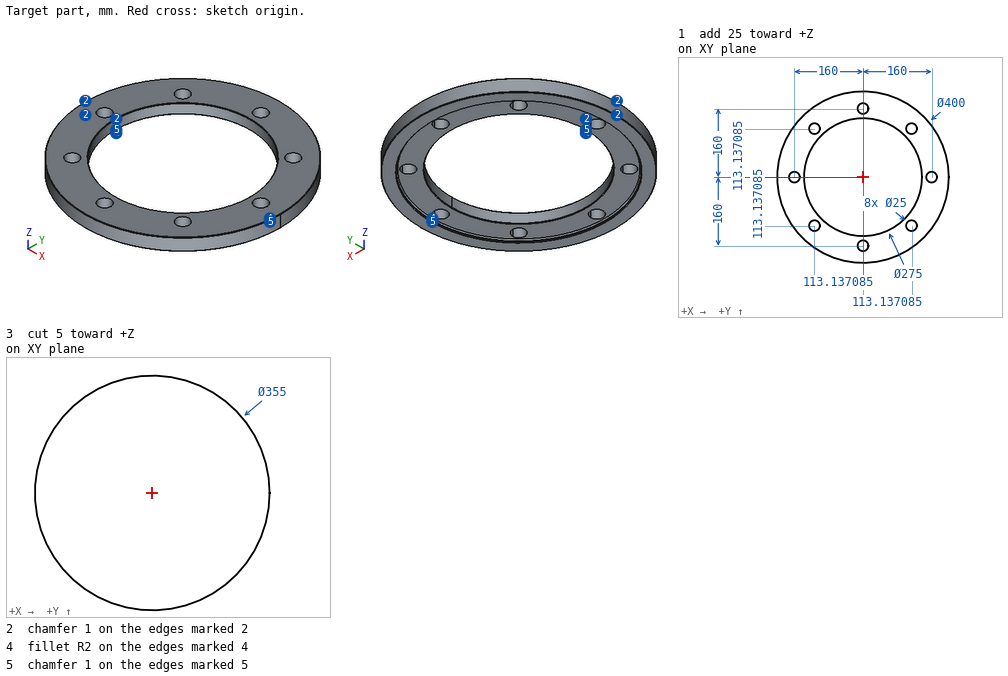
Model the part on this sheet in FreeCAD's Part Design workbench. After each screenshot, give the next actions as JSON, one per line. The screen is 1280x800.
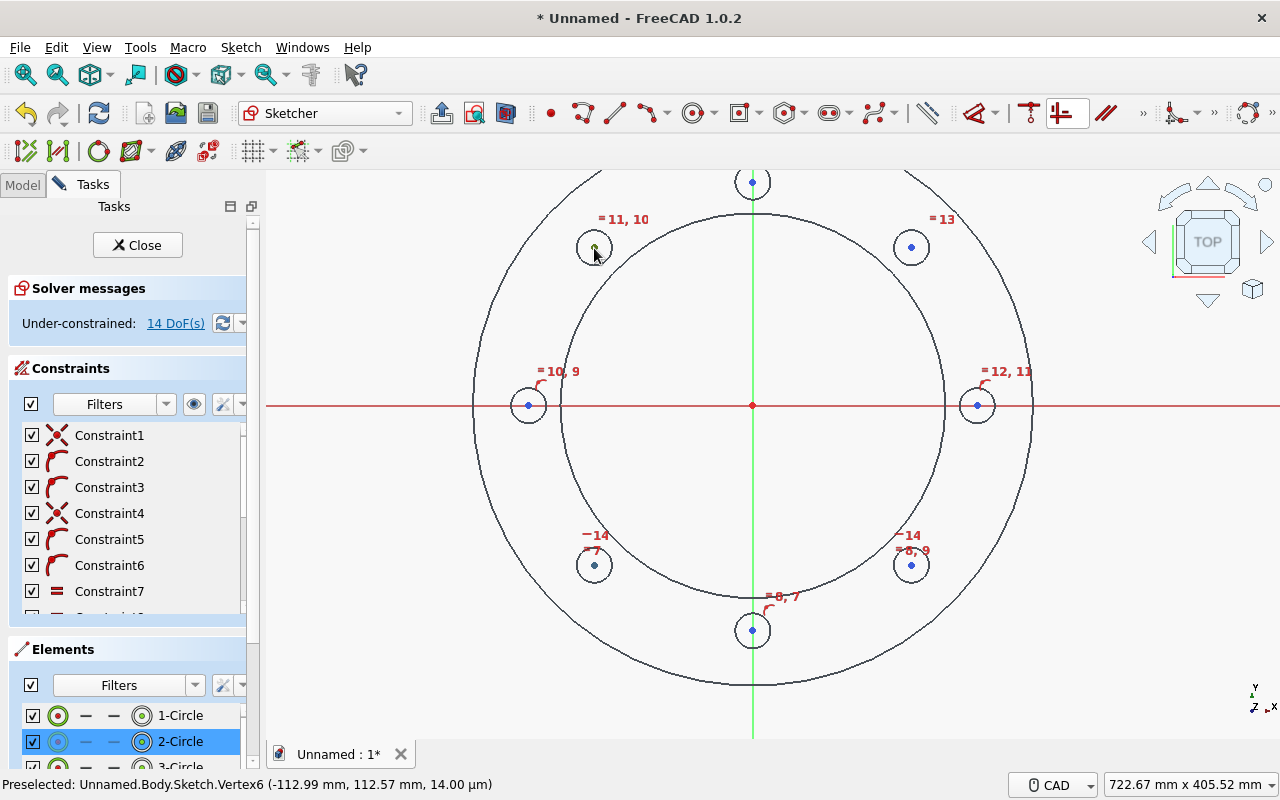
{"action": "left_click", "coordinate": [1084, 114]}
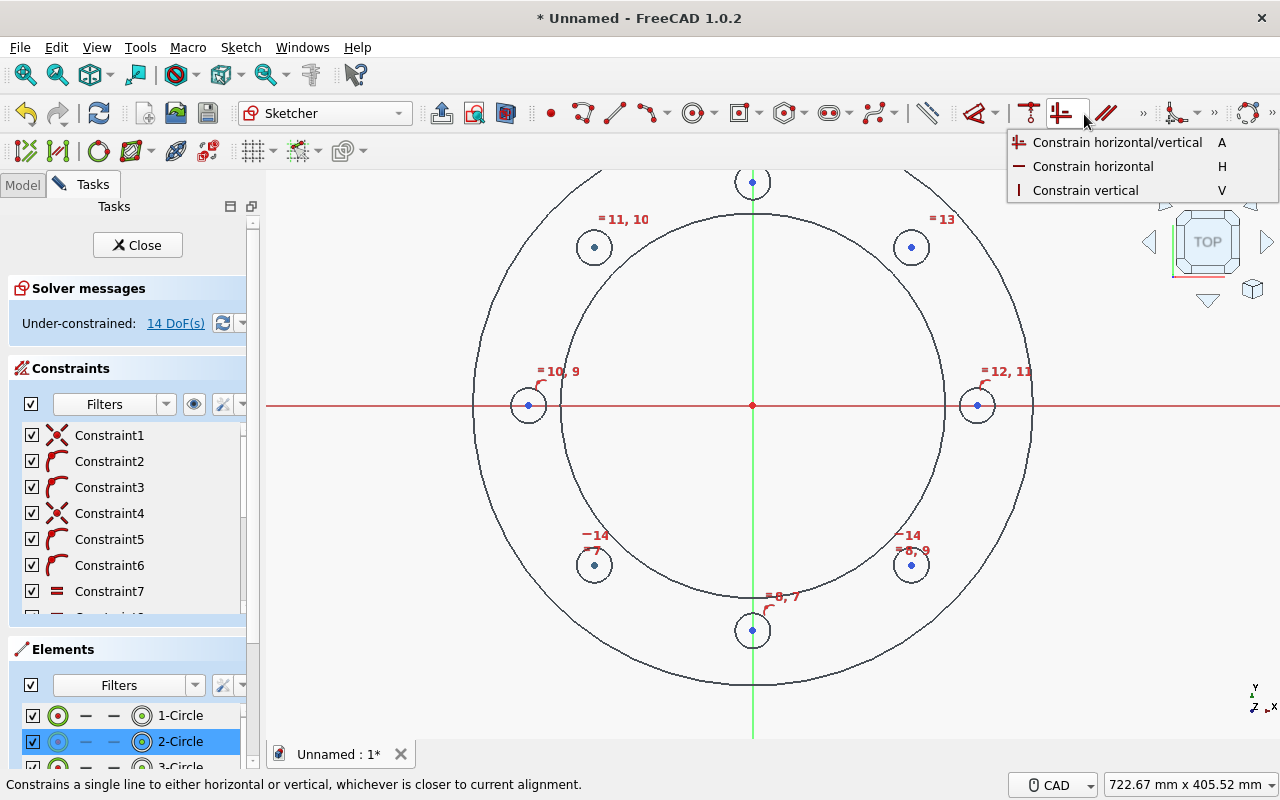
{"action": "left_click", "coordinate": [1143, 190]}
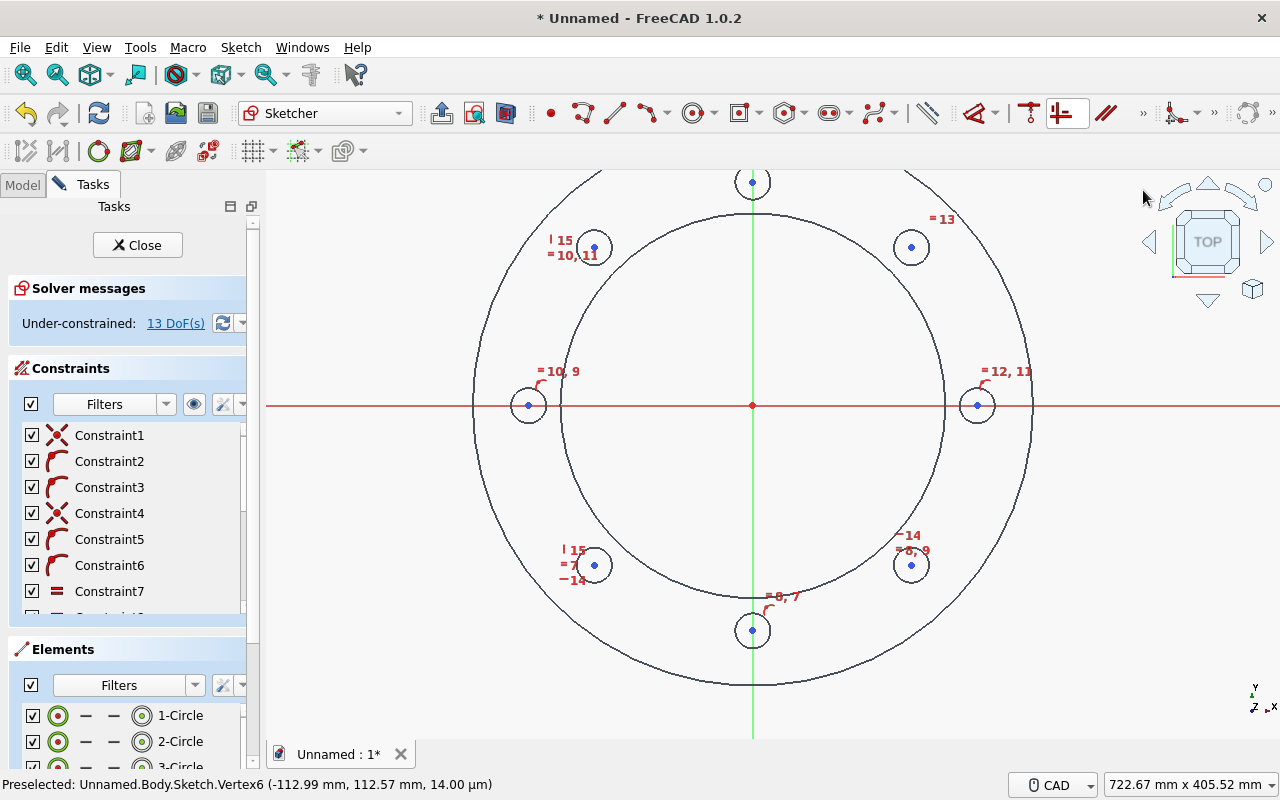
{"action": "left_click", "coordinate": [911, 565]}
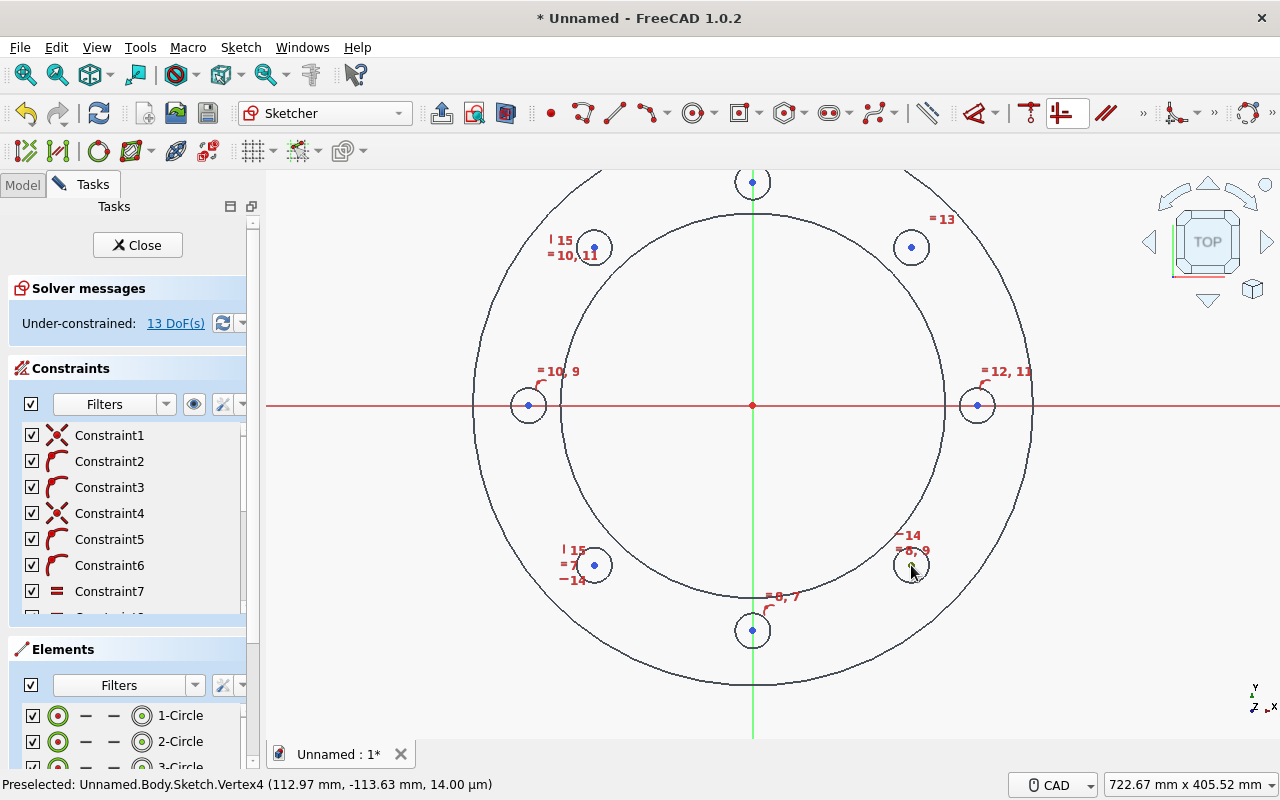
{"action": "left_click", "coordinate": [912, 248]}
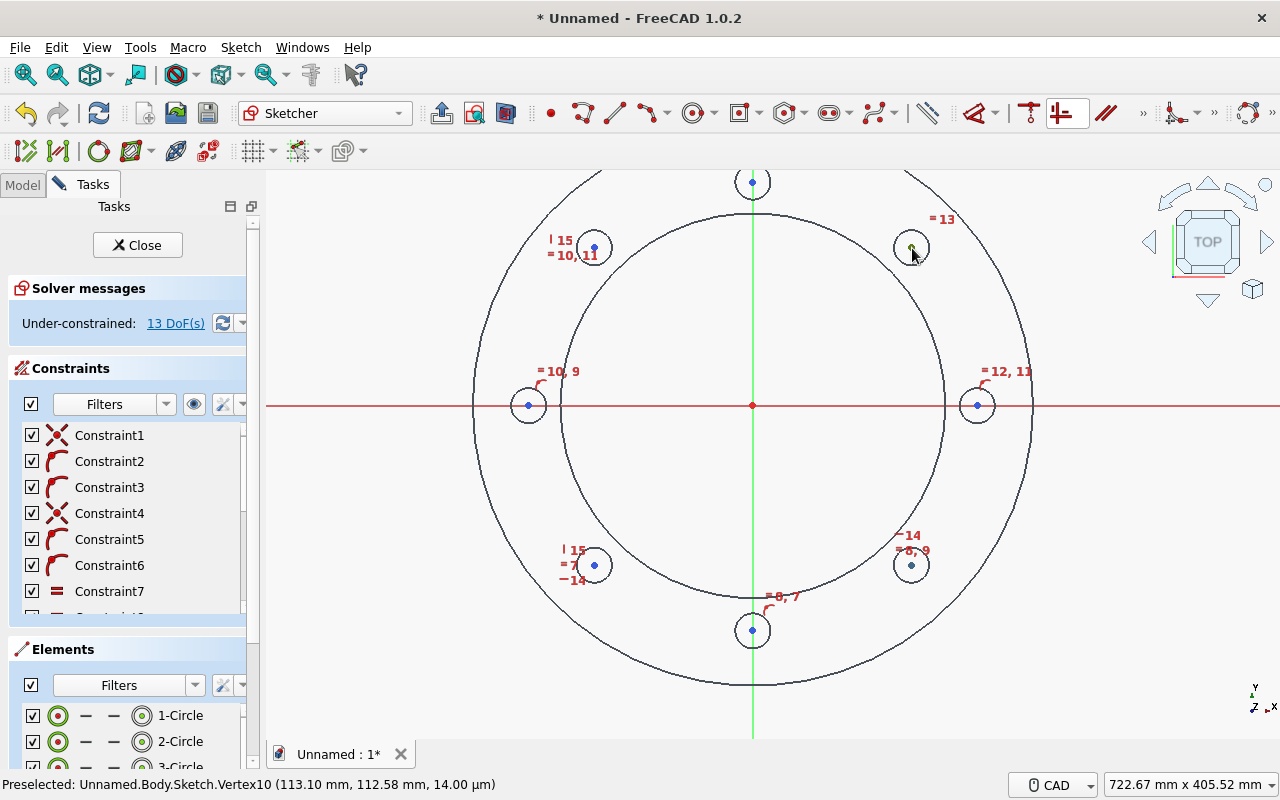
{"action": "left_click", "coordinate": [1084, 114]}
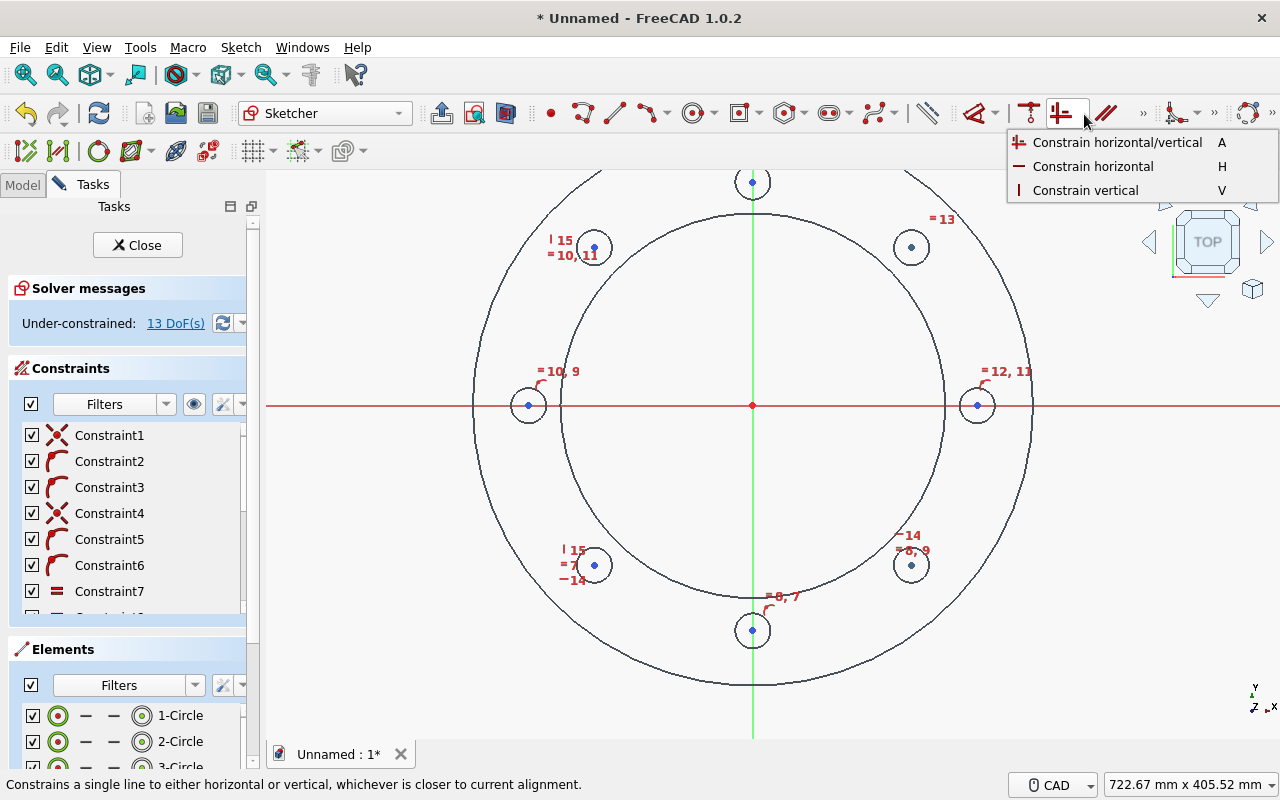
{"action": "left_click", "coordinate": [1143, 190]}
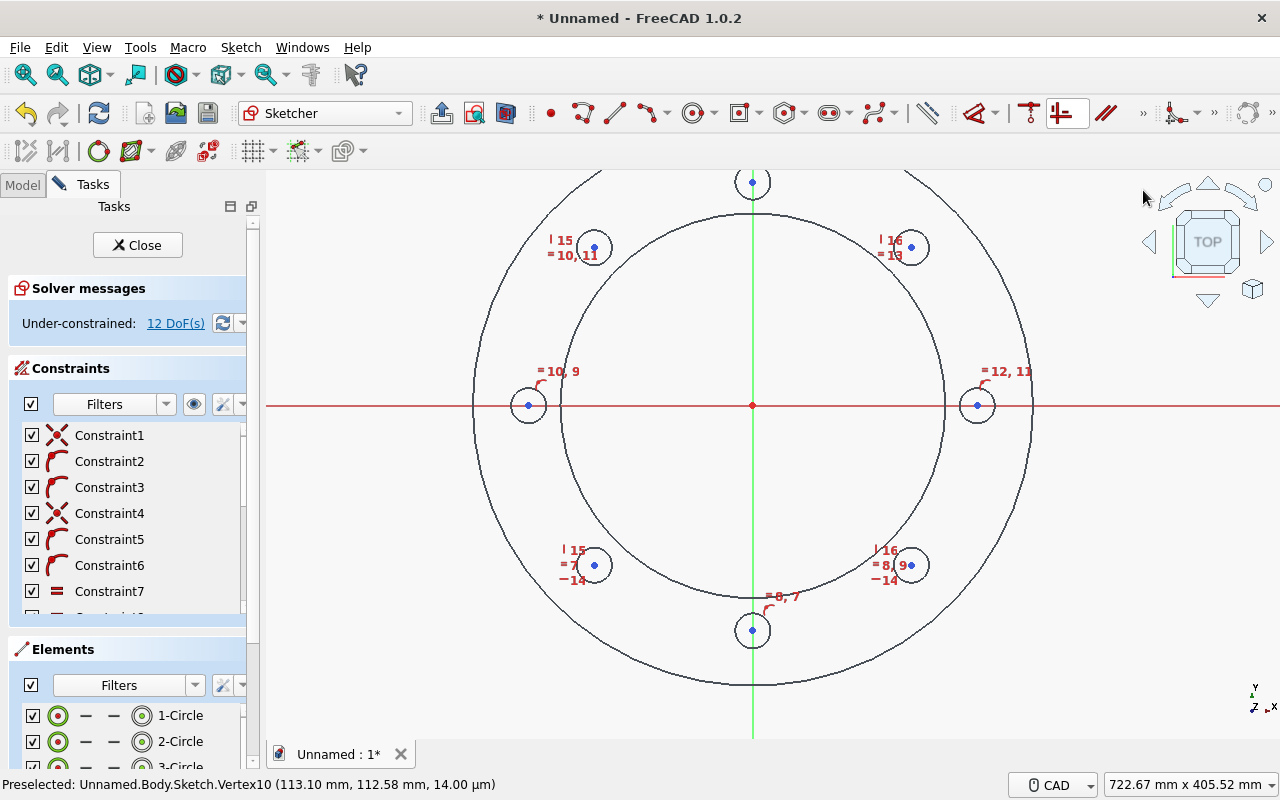
{"action": "scroll", "coordinate": [594, 248], "scroll_direction": "up", "scroll_amount": 4}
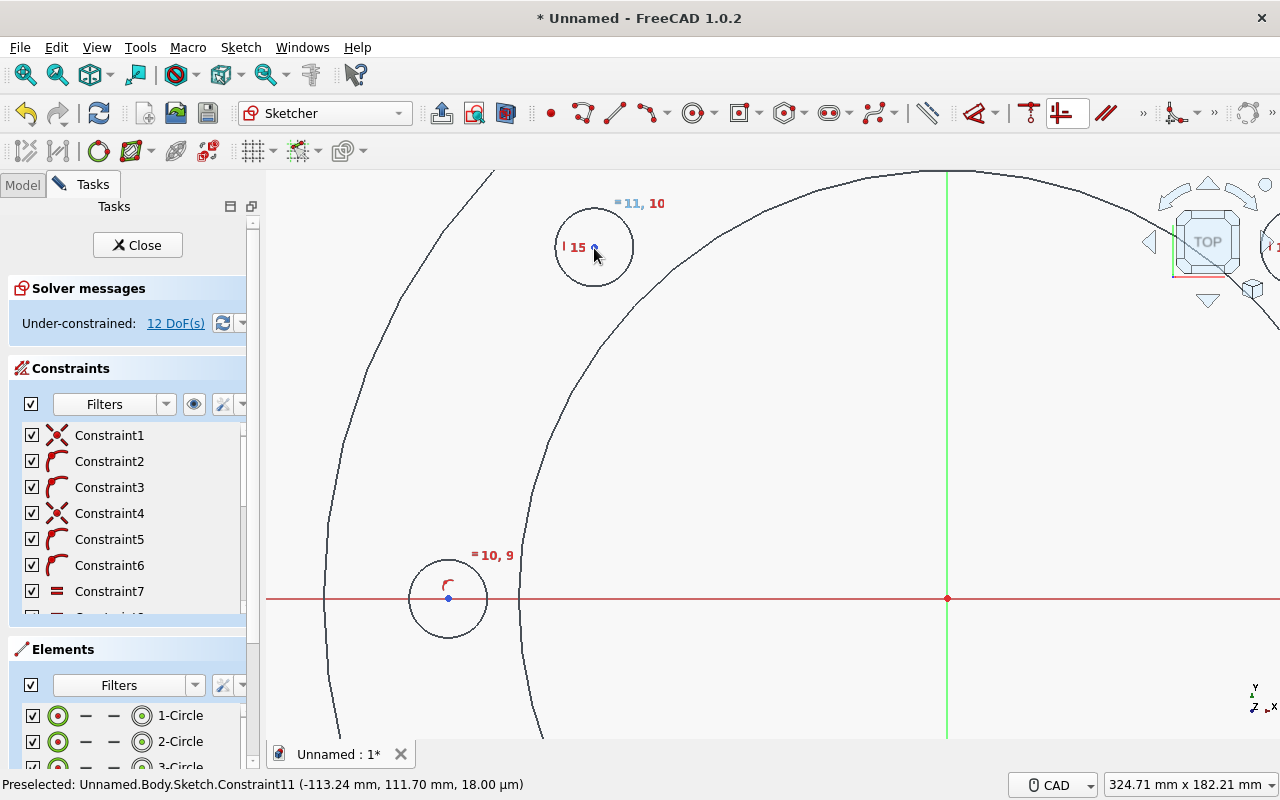
{"action": "left_click", "coordinate": [594, 247]}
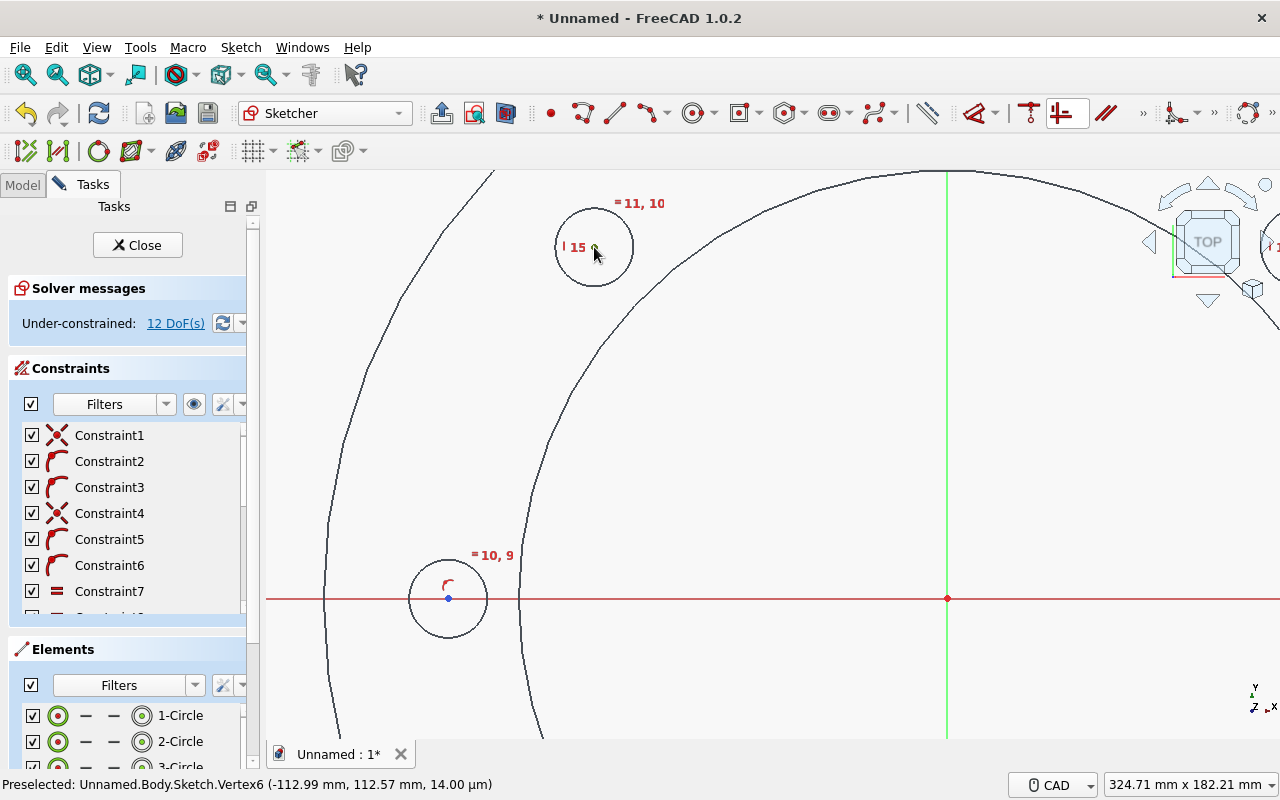
{"action": "scroll", "coordinate": [600, 392], "scroll_direction": "down", "scroll_amount": 6}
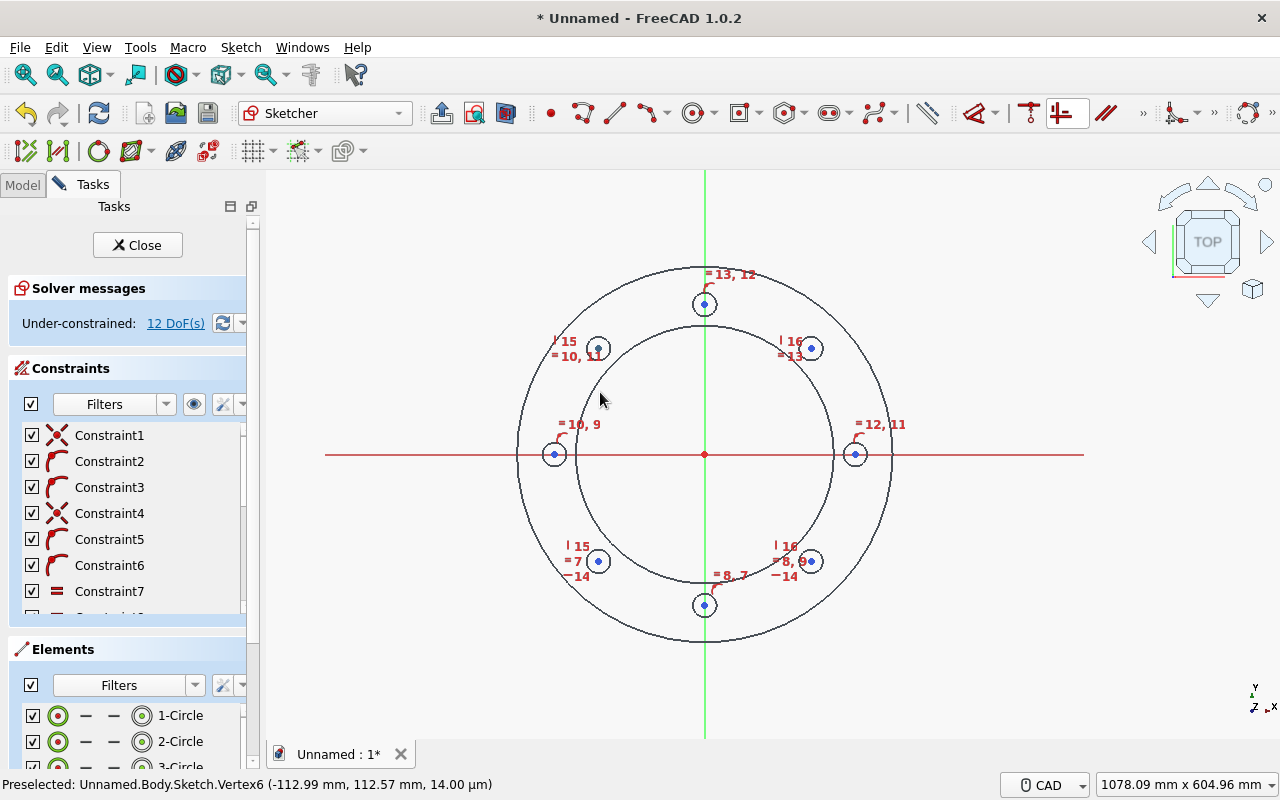
{"action": "left_click", "coordinate": [811, 349]}